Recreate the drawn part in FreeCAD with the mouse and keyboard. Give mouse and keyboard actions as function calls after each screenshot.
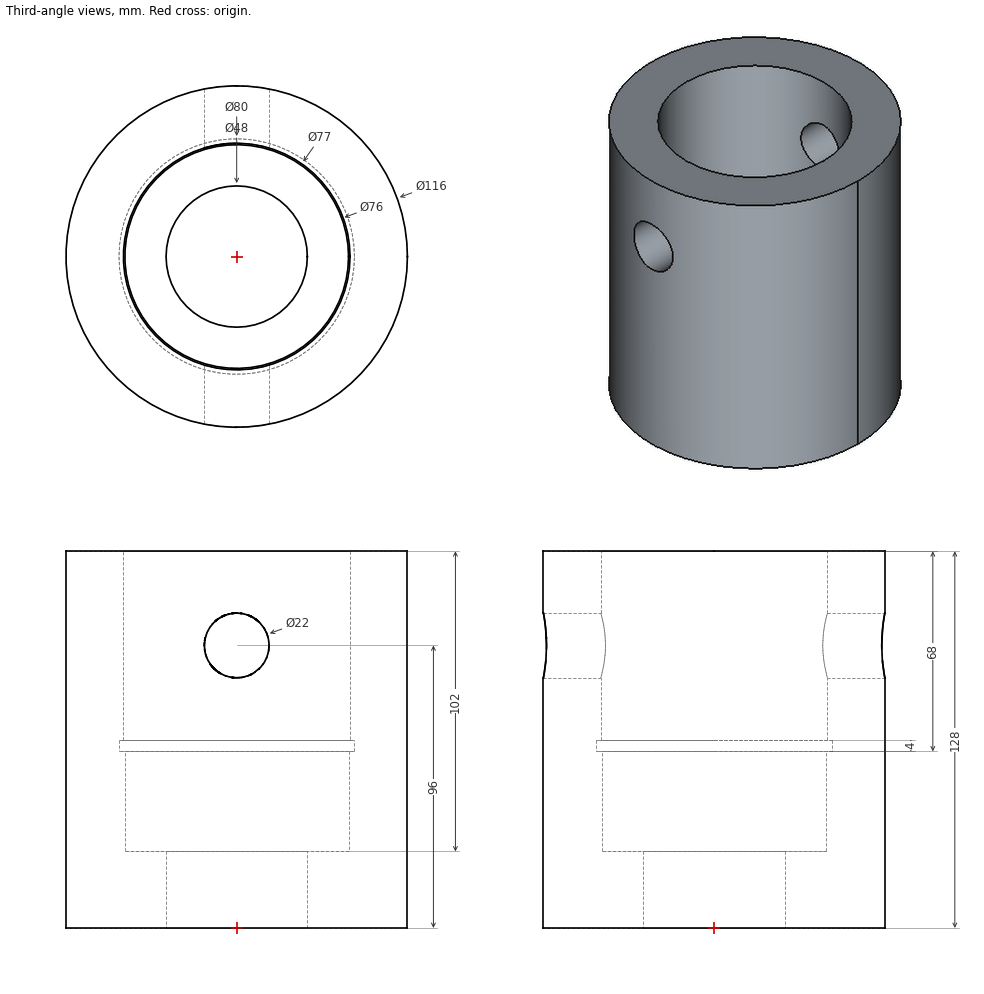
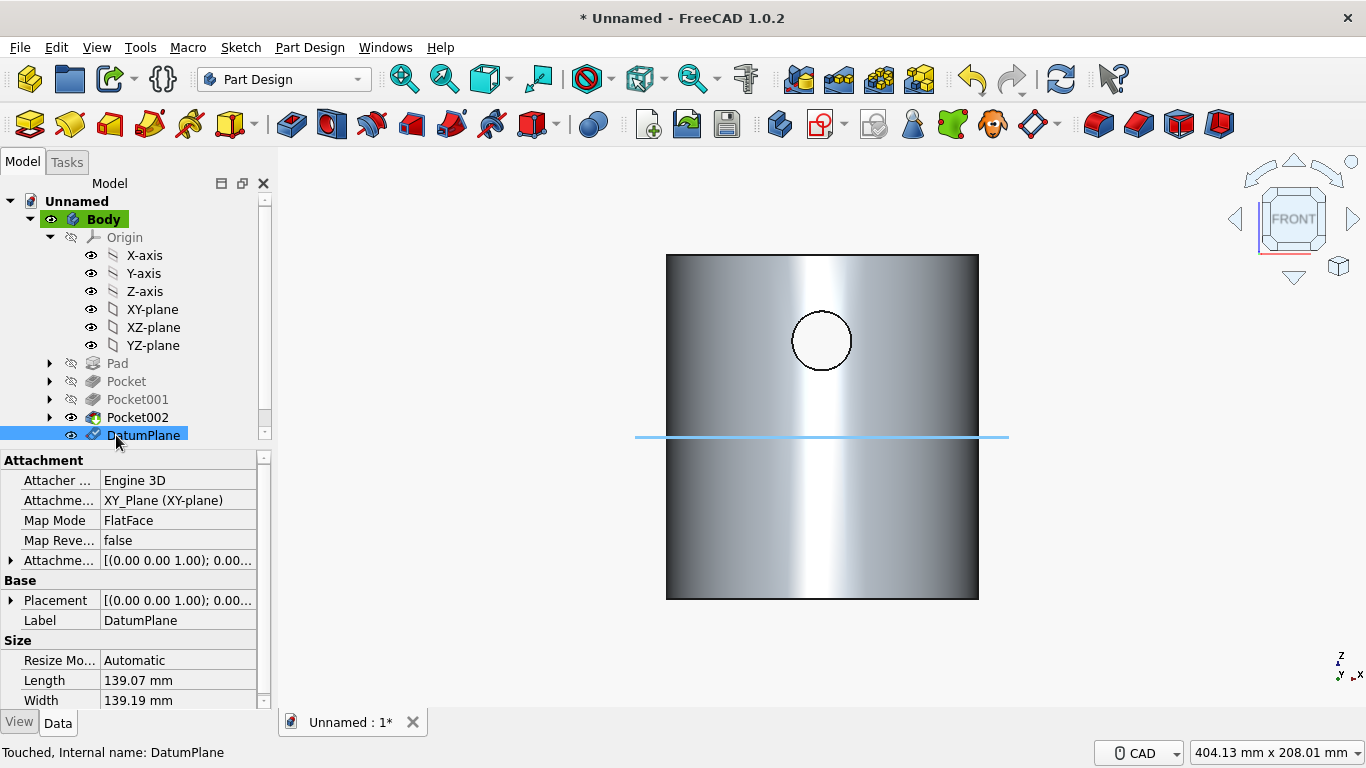
click(820, 124)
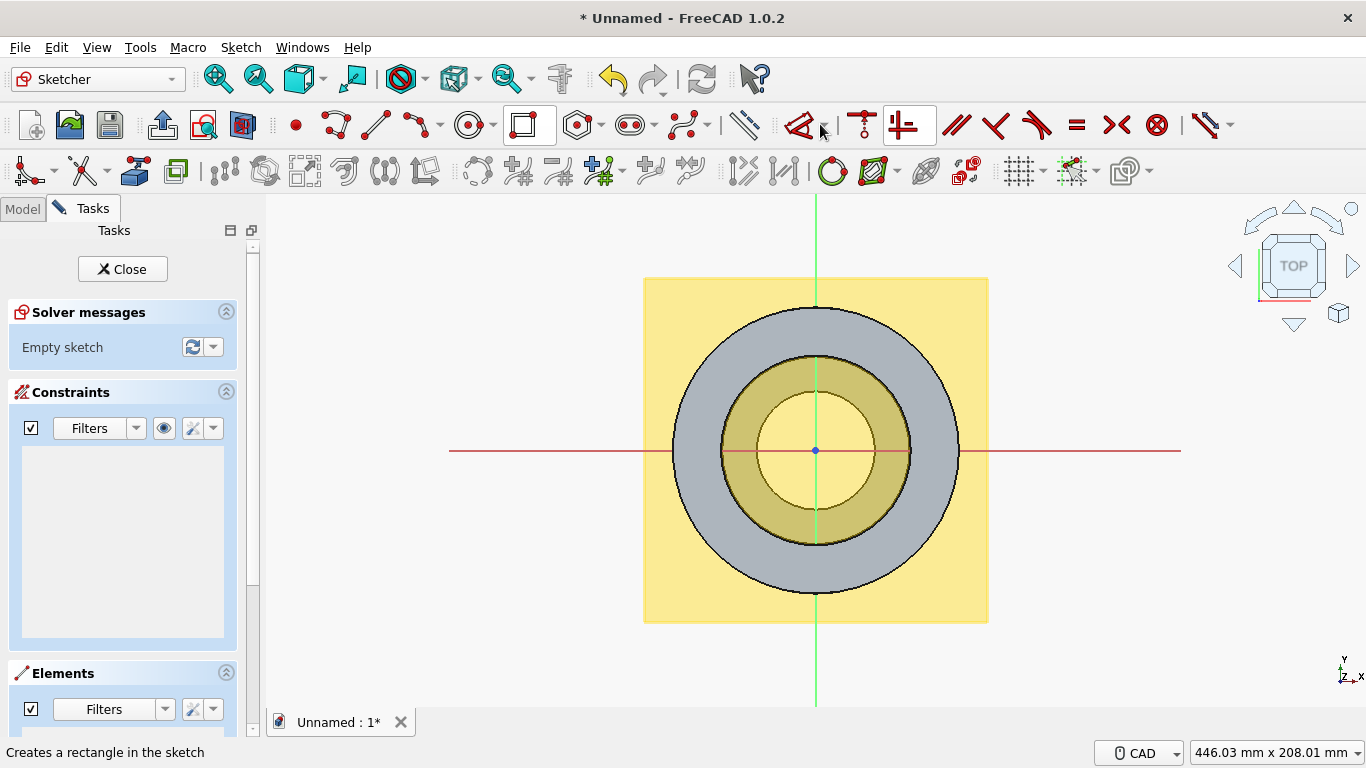
click(244, 126)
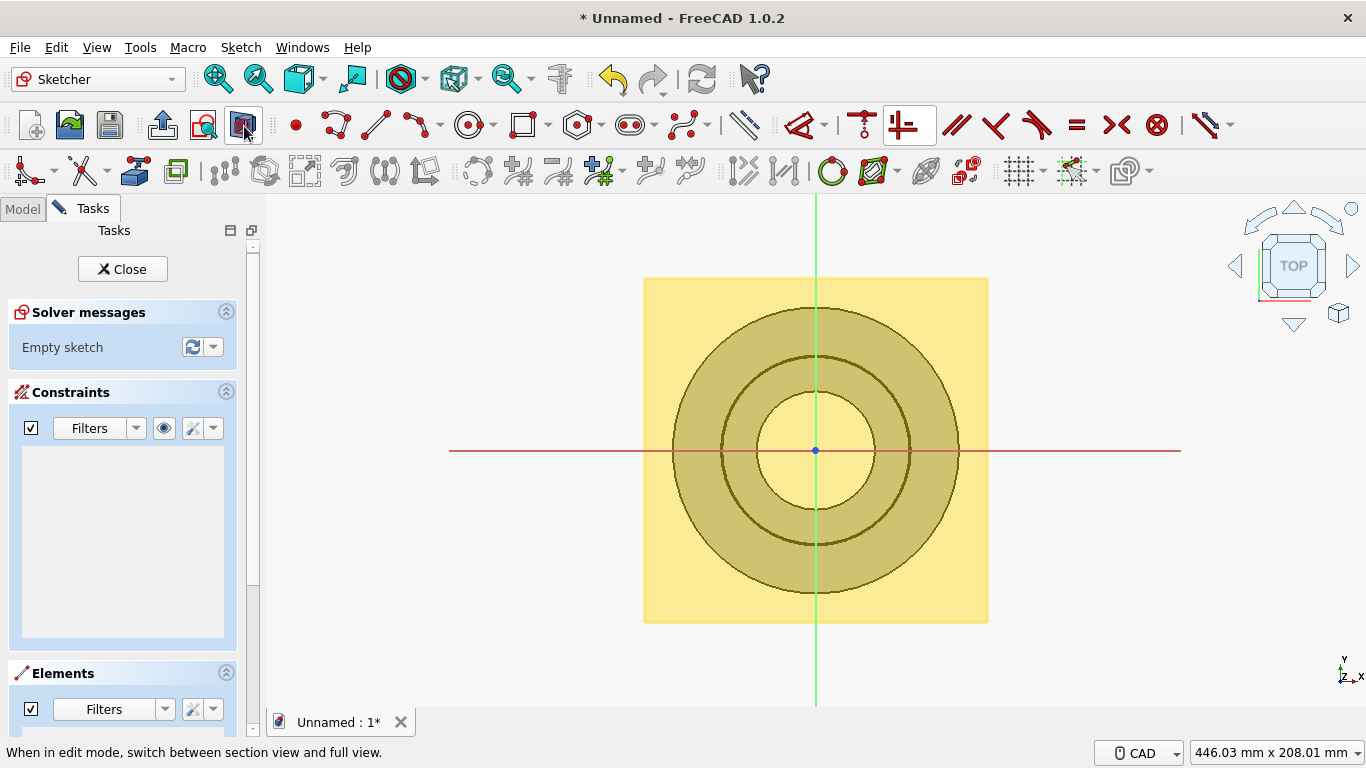
scroll(955, 450, up, 2)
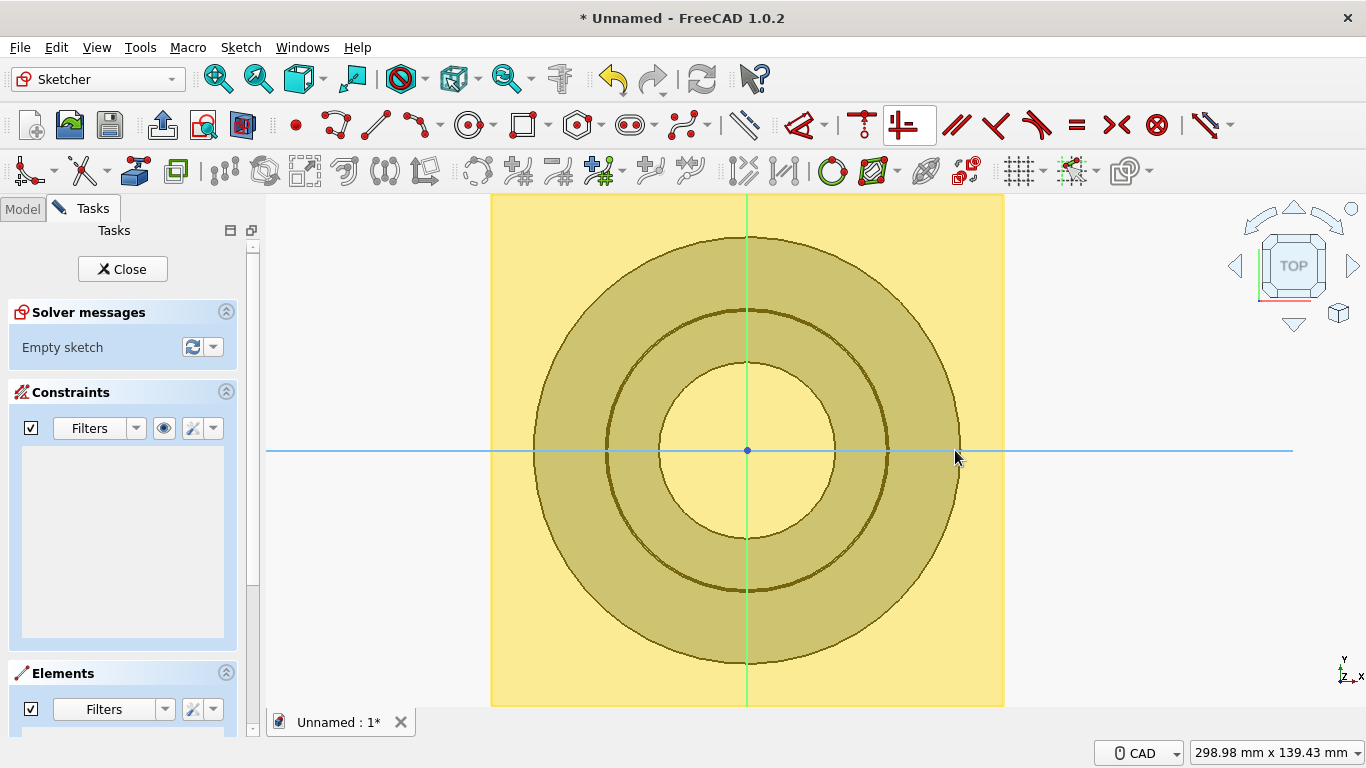
click(470, 126)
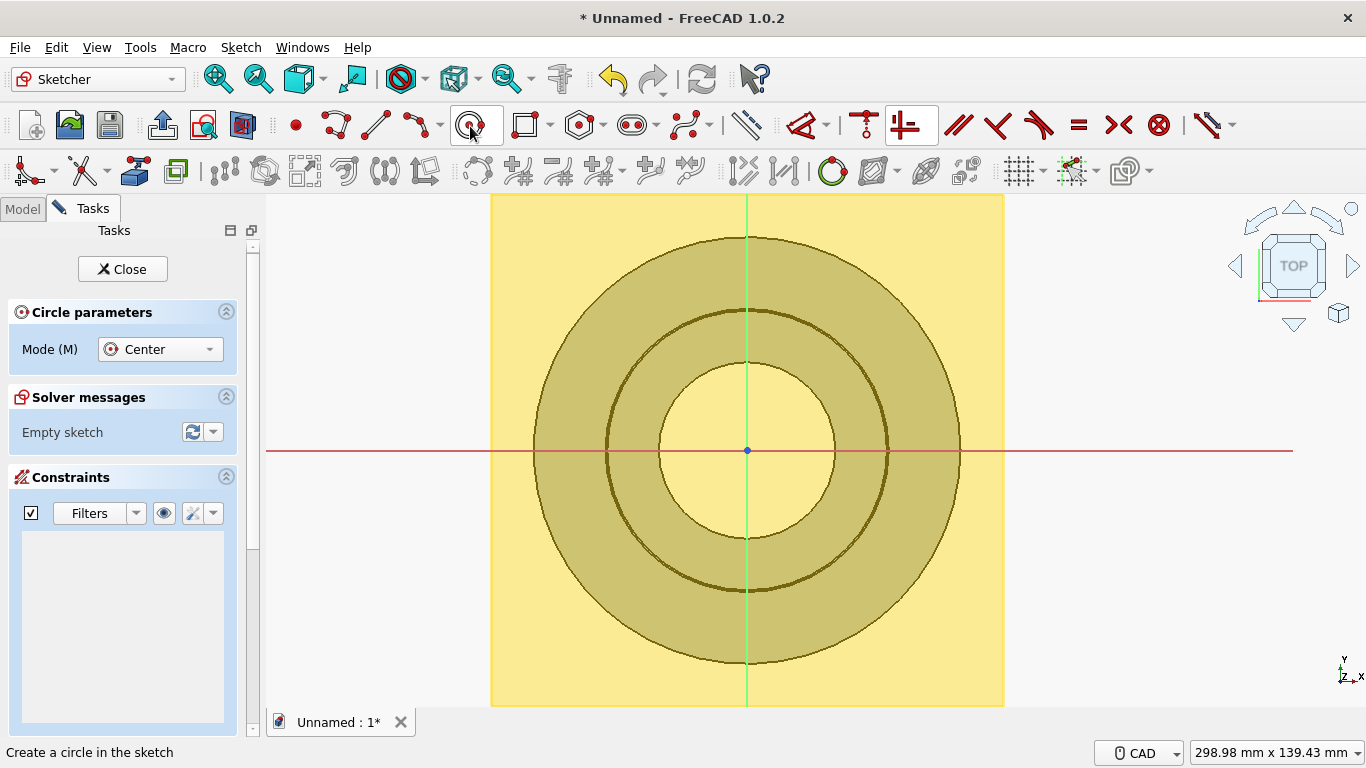
click(747, 450)
move(851, 346)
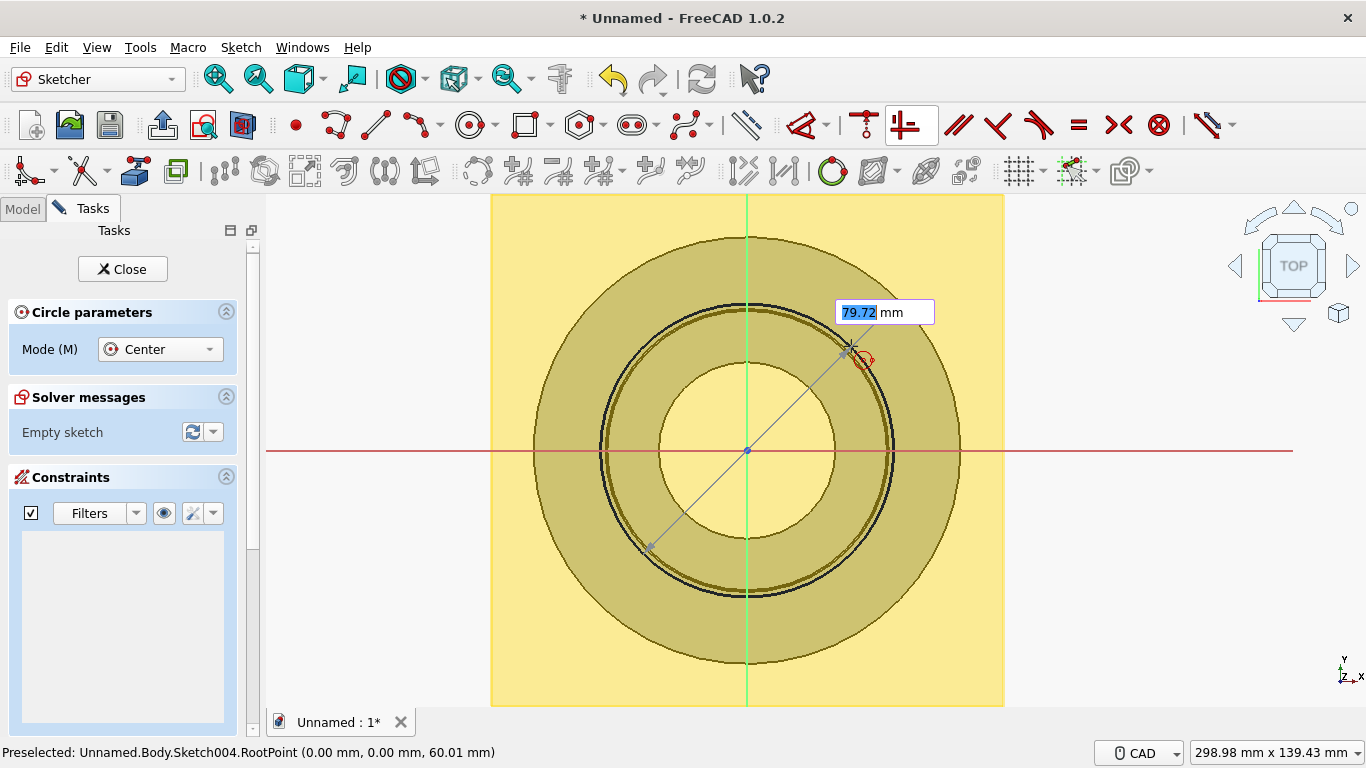
text(80)
key(Return)
key(Escape)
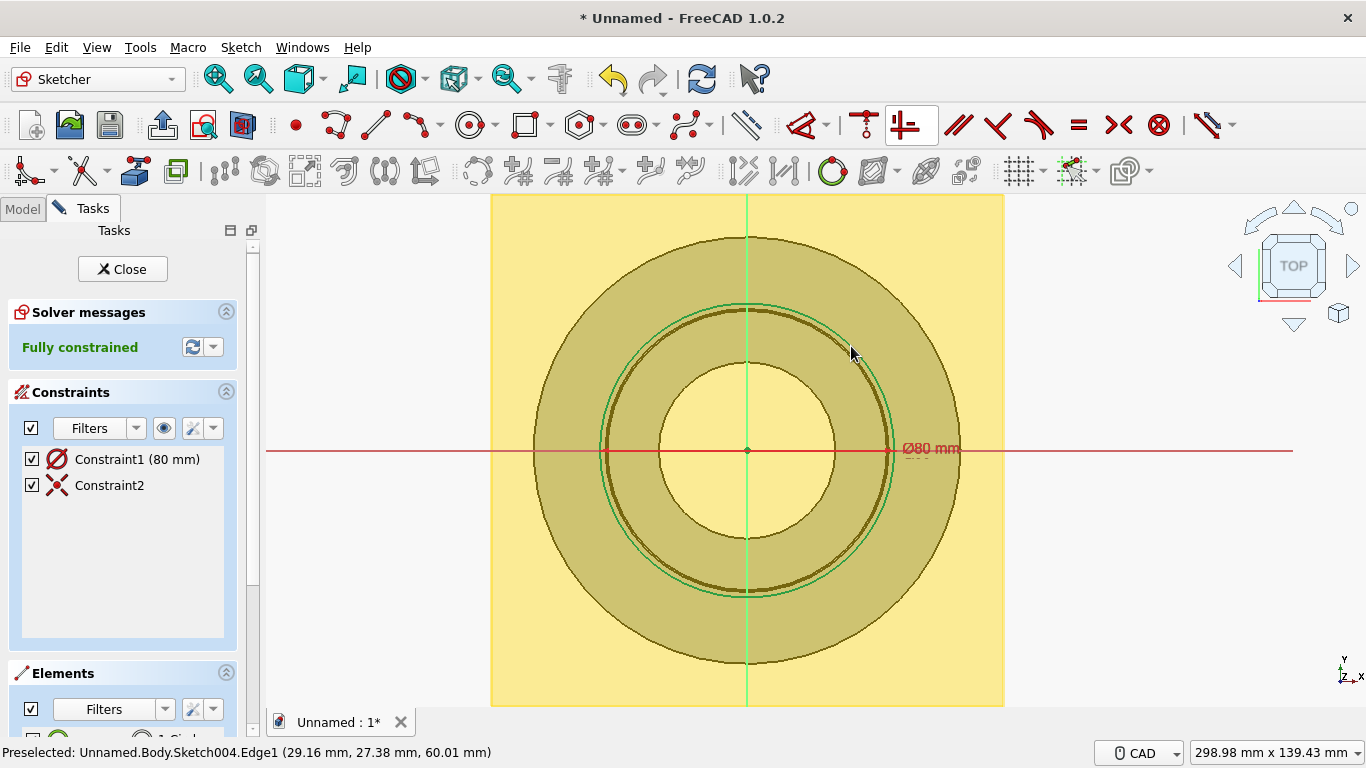
click(123, 269)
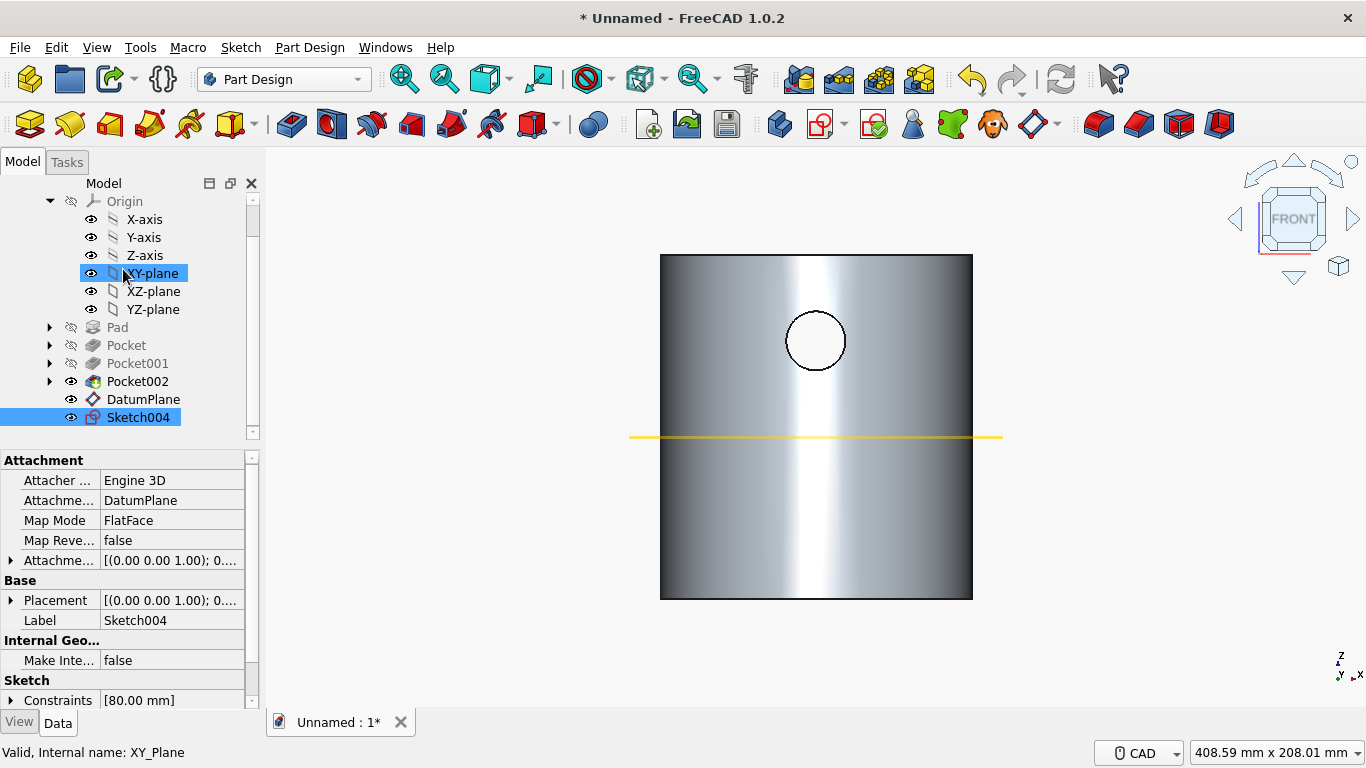
click(292, 124)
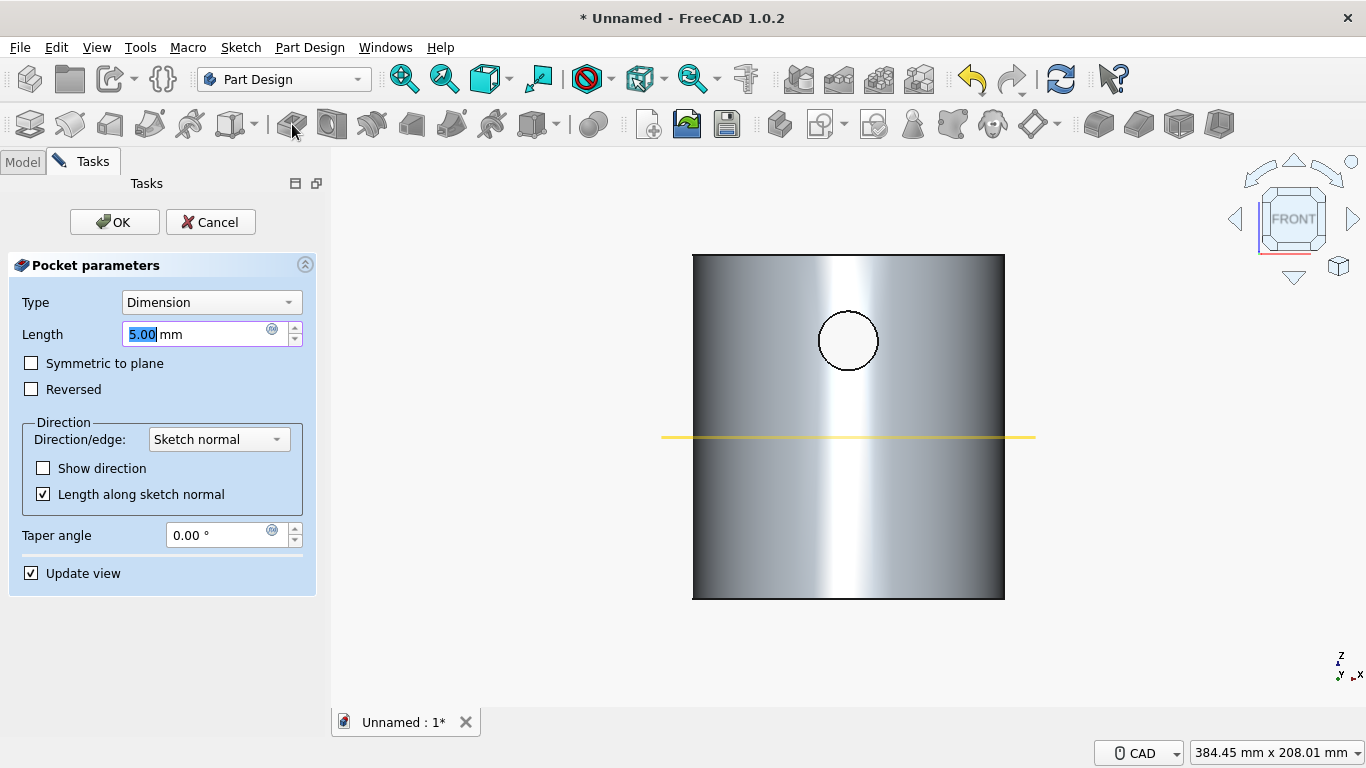
text(4)
key(Tab)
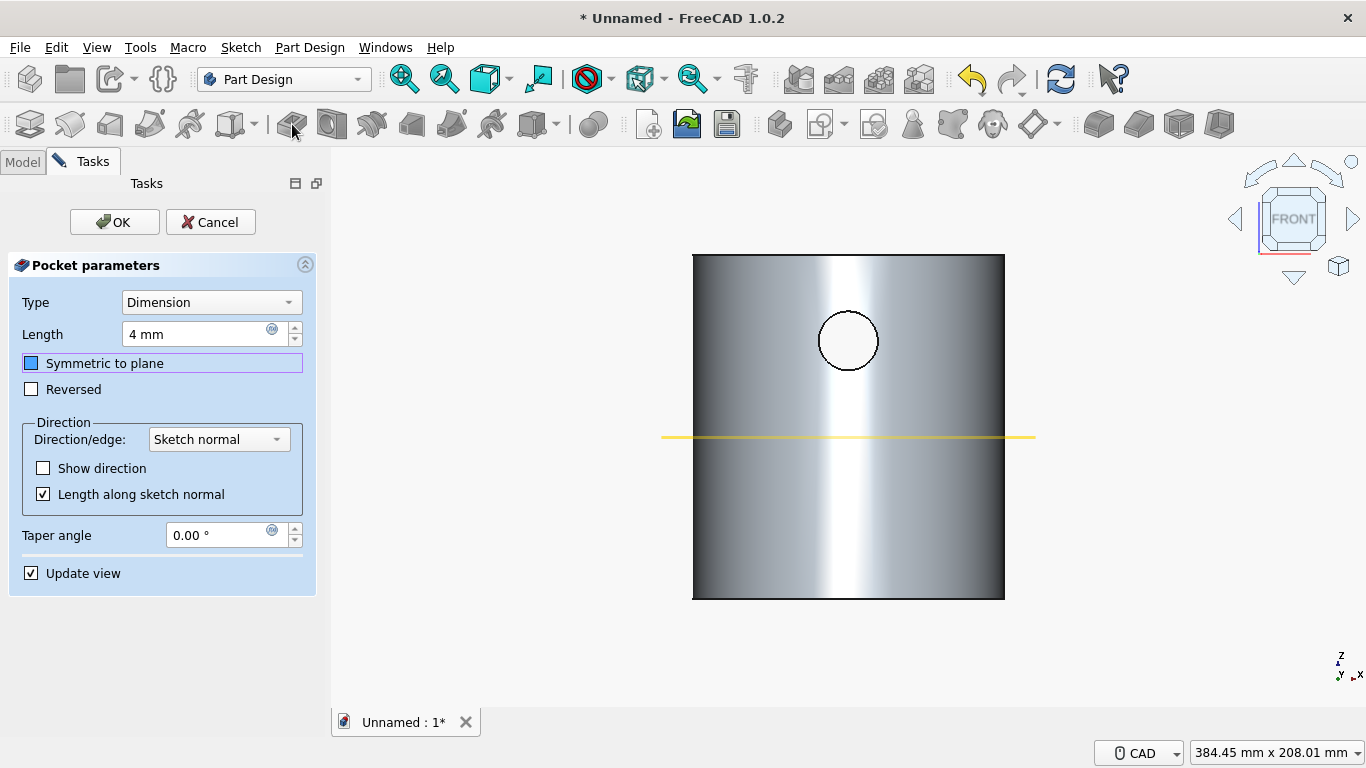
click(30, 389)